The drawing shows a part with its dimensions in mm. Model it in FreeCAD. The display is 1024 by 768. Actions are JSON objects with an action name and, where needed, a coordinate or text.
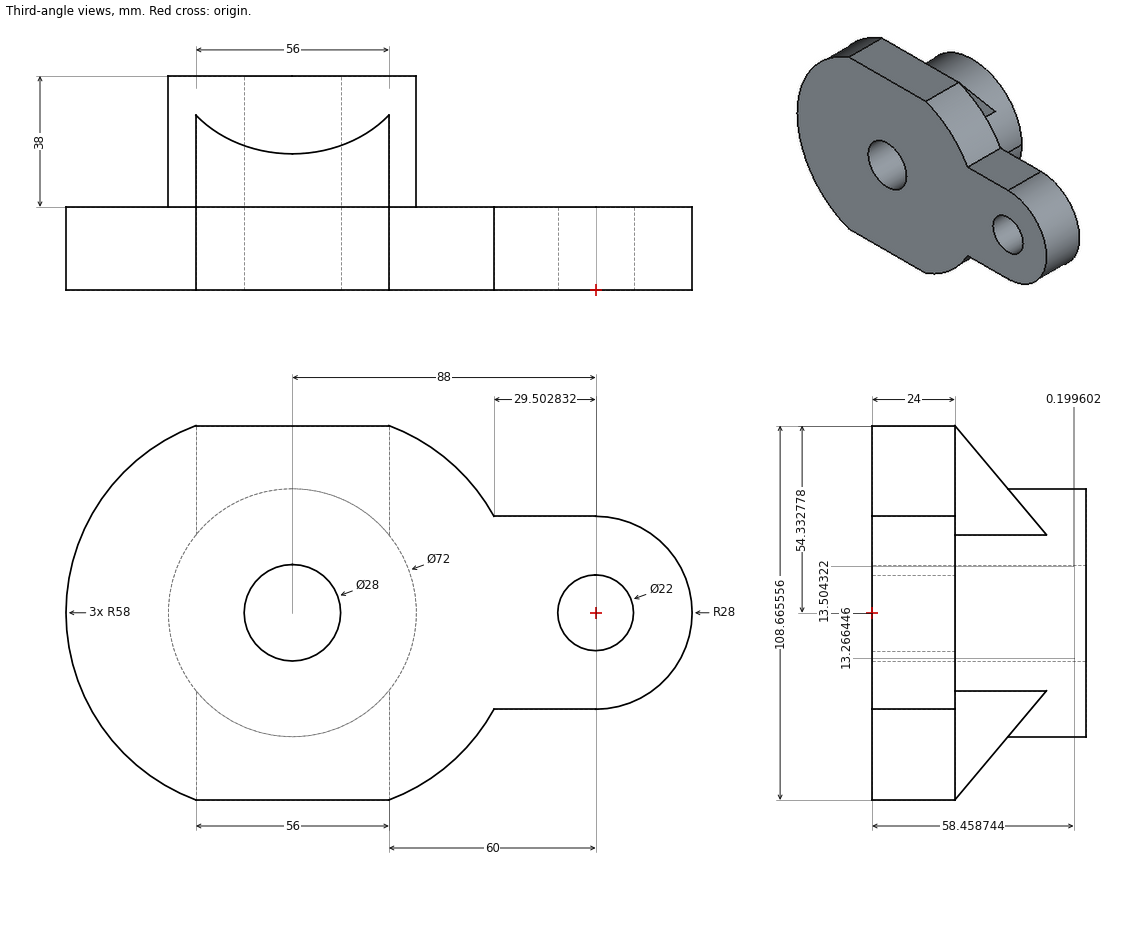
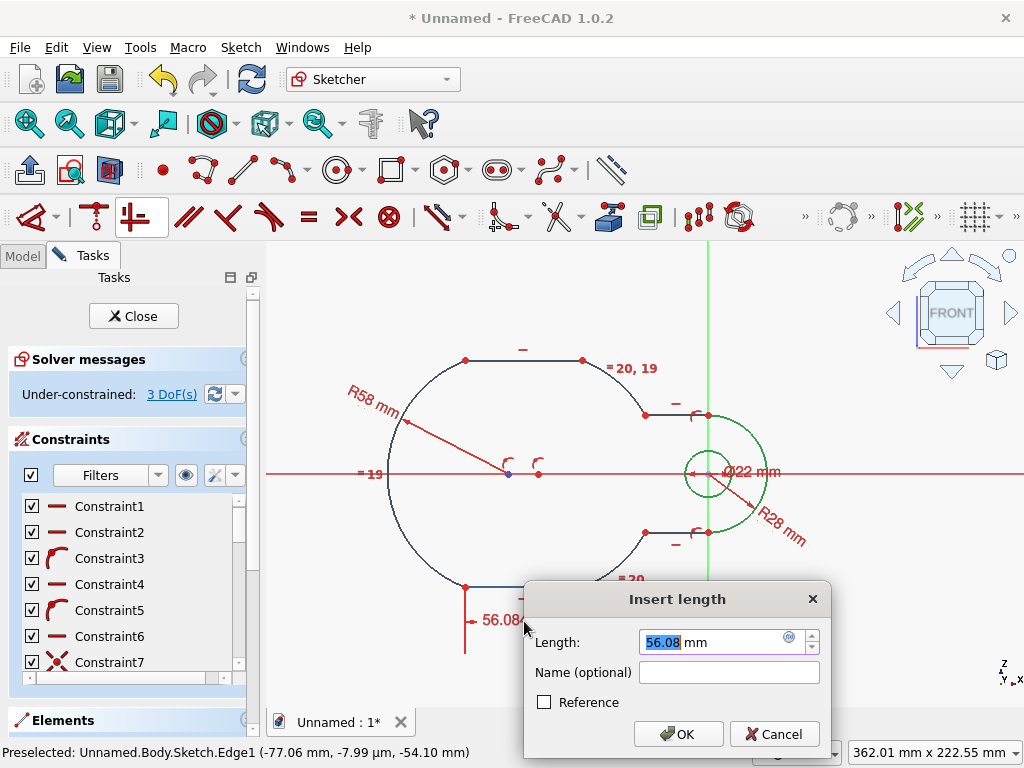
{"action": "type", "text": "56"}
{"action": "key", "text": "Return"}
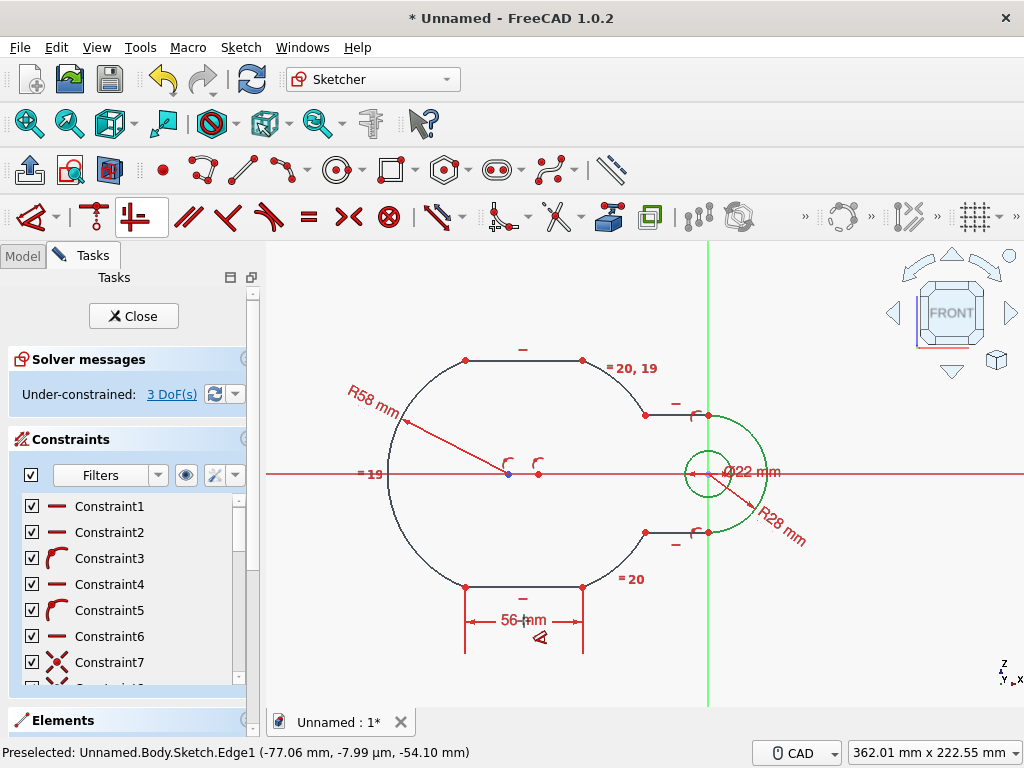
{"action": "left_click", "coordinate": [500, 361]}
{"action": "left_click", "coordinate": [524, 327]}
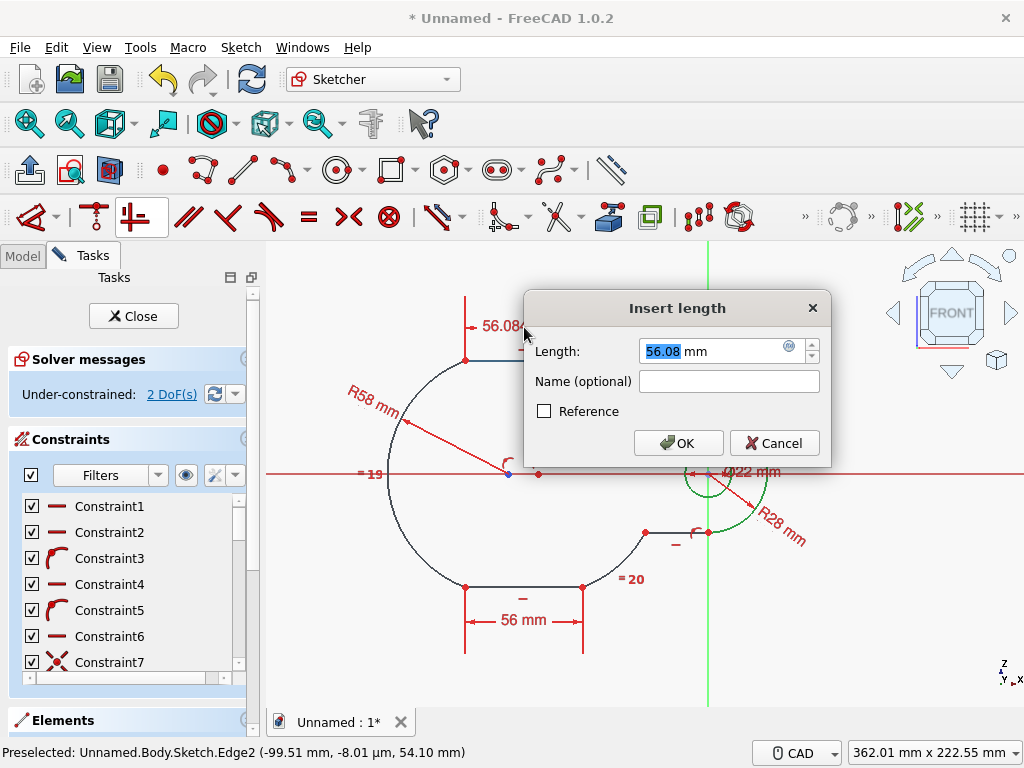
{"action": "type", "text": "56"}
{"action": "key", "text": "Return"}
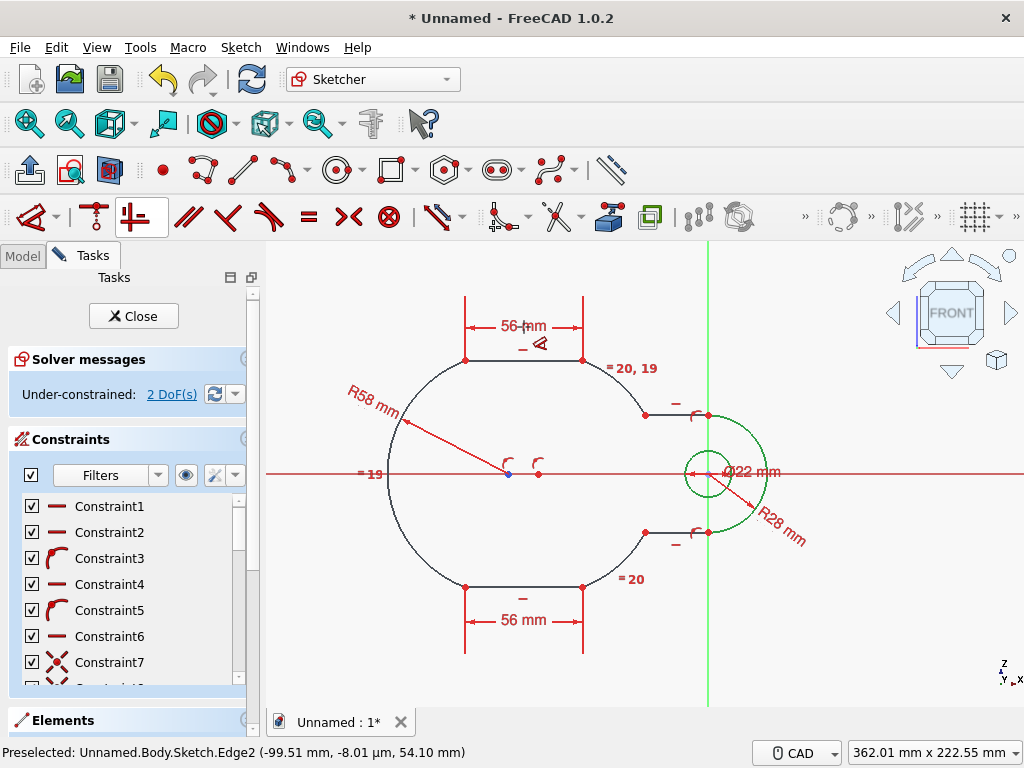
{"action": "left_click", "coordinate": [583, 587]}
{"action": "left_click", "coordinate": [645, 621]}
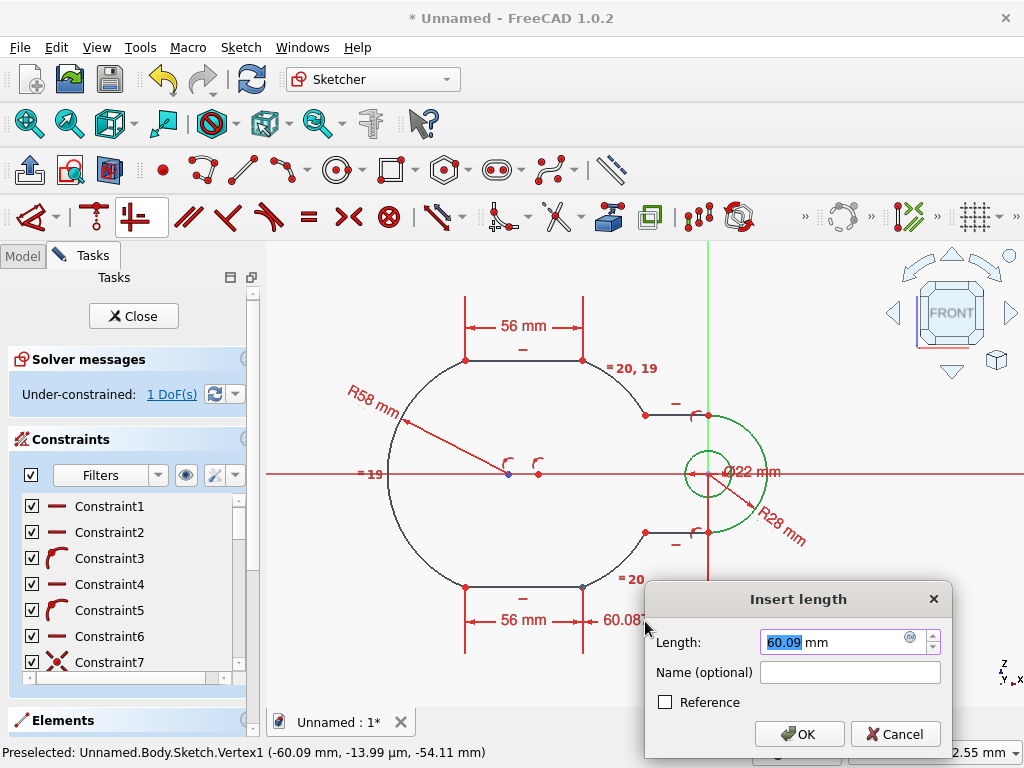
{"action": "type", "text": "60"}
{"action": "key", "text": "Return"}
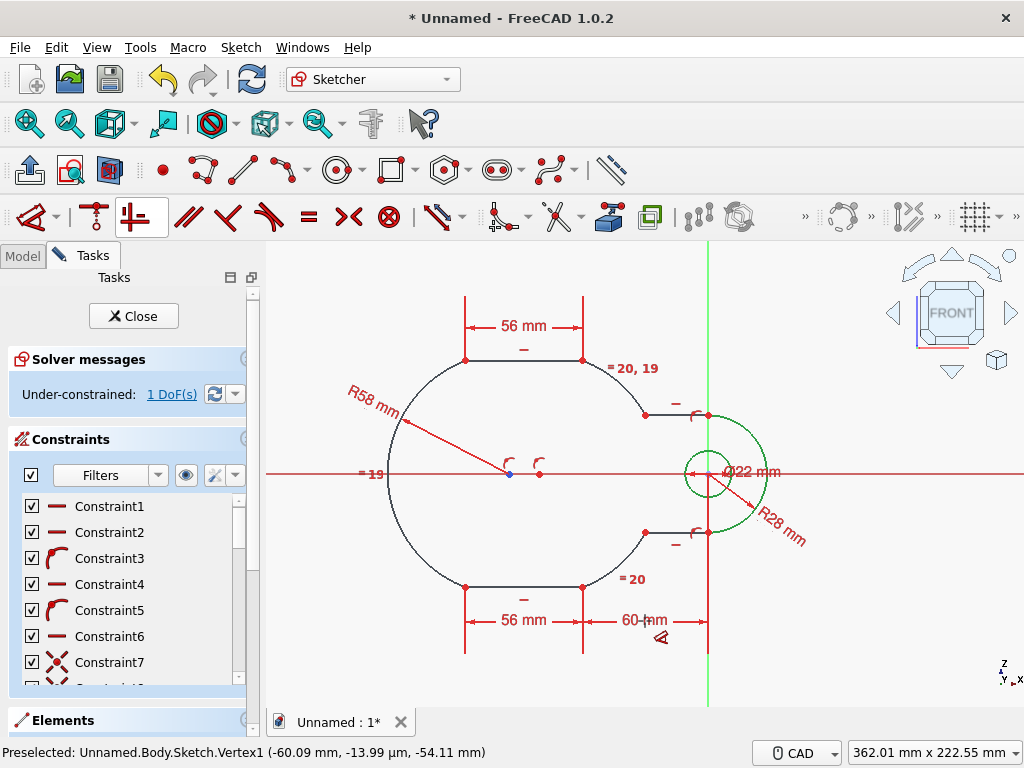
{"action": "left_click", "coordinate": [664, 415]}
{"action": "left_click", "coordinate": [677, 381]}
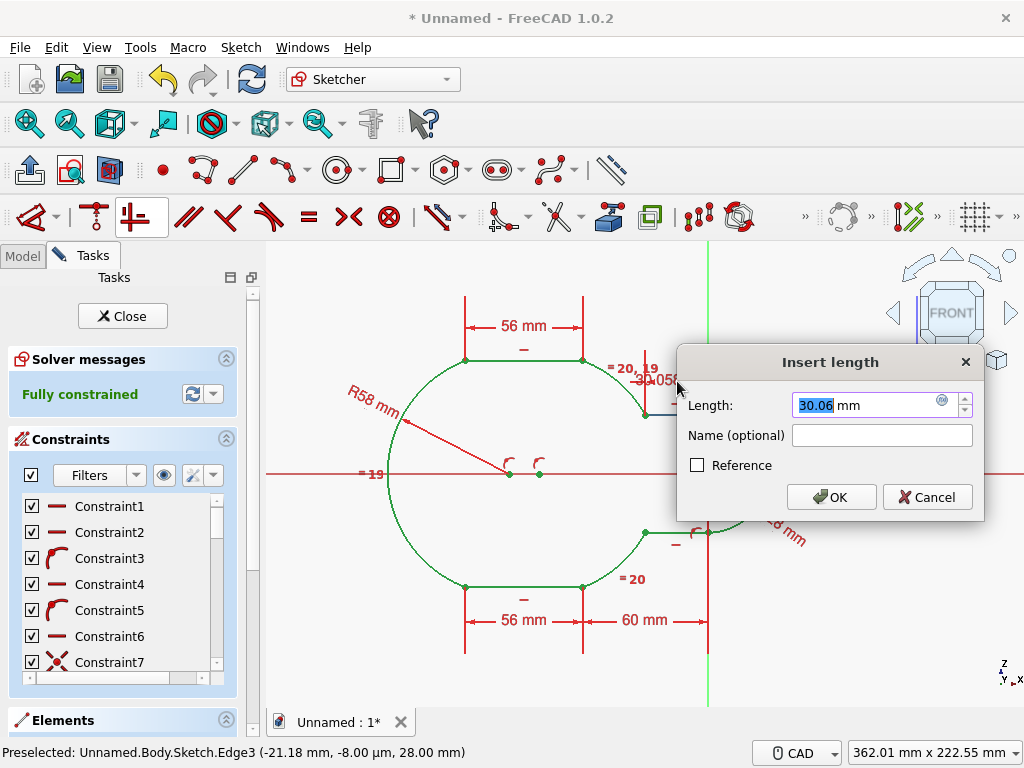
{"action": "type", "text": "29.502832"}
{"action": "key", "text": "Return"}
{"action": "key", "text": "Escape"}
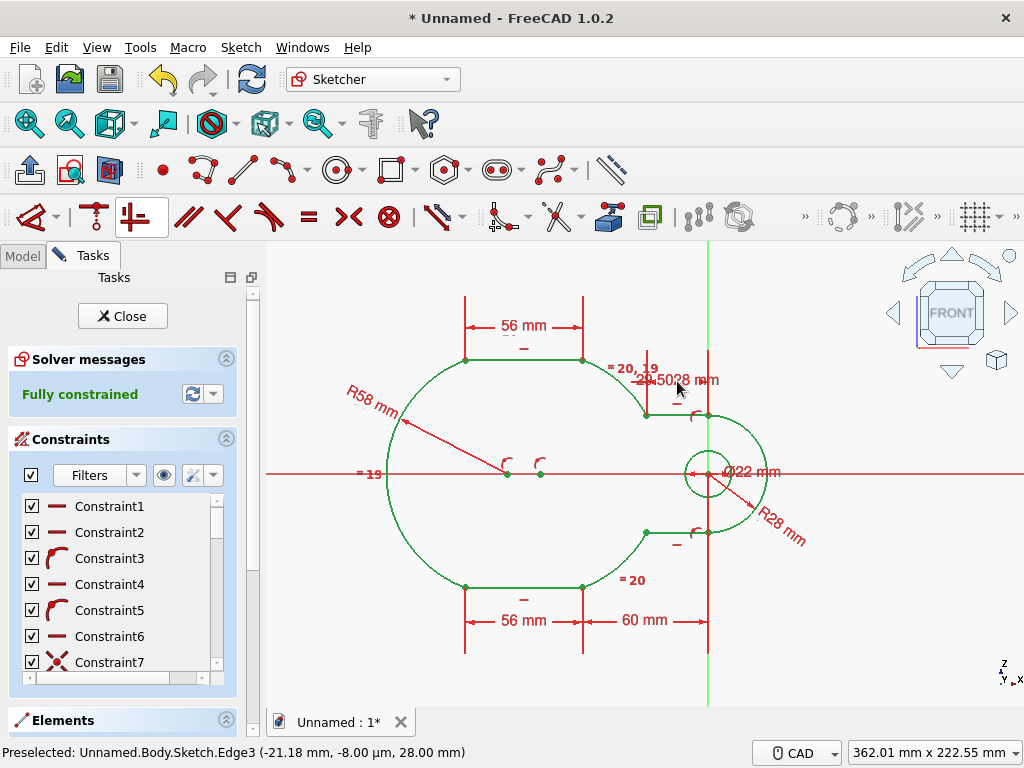
{"action": "left_click", "coordinate": [123, 316]}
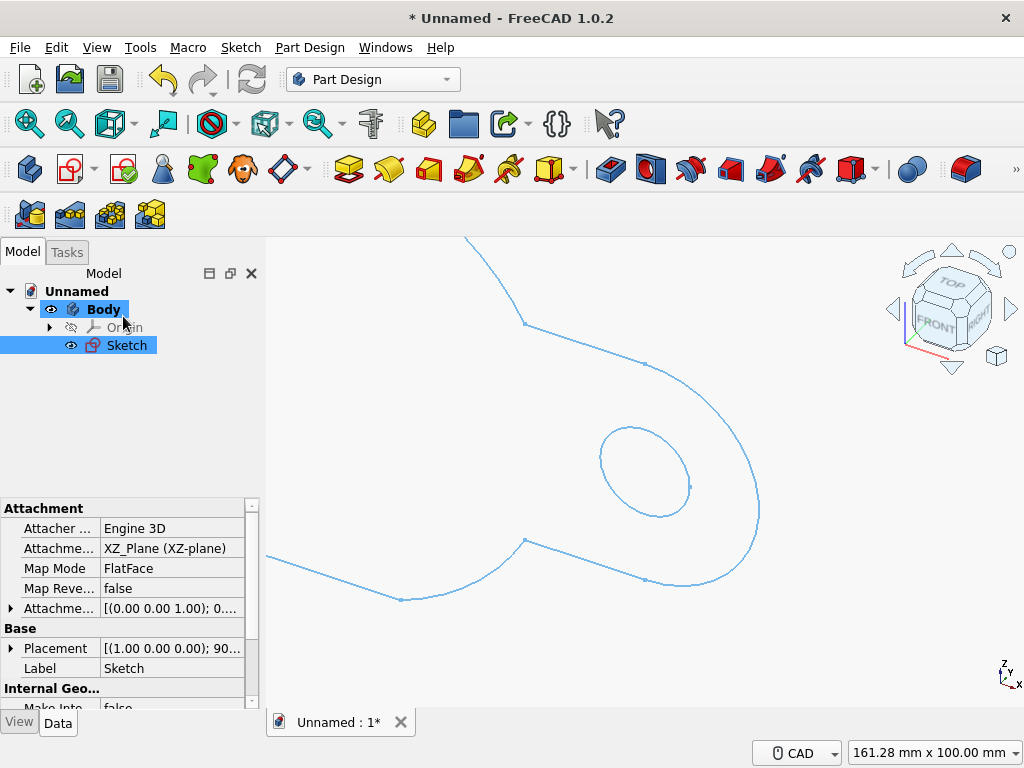
{"action": "left_click", "coordinate": [350, 170]}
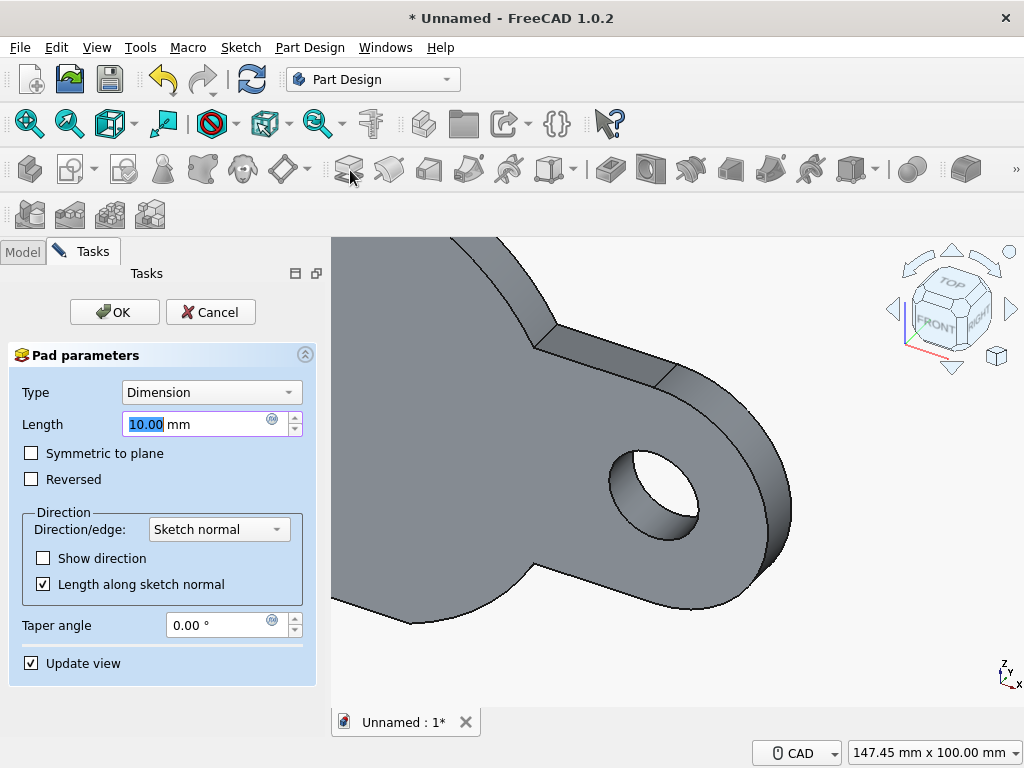
{"action": "type", "text": "24"}
{"action": "key", "text": "Tab"}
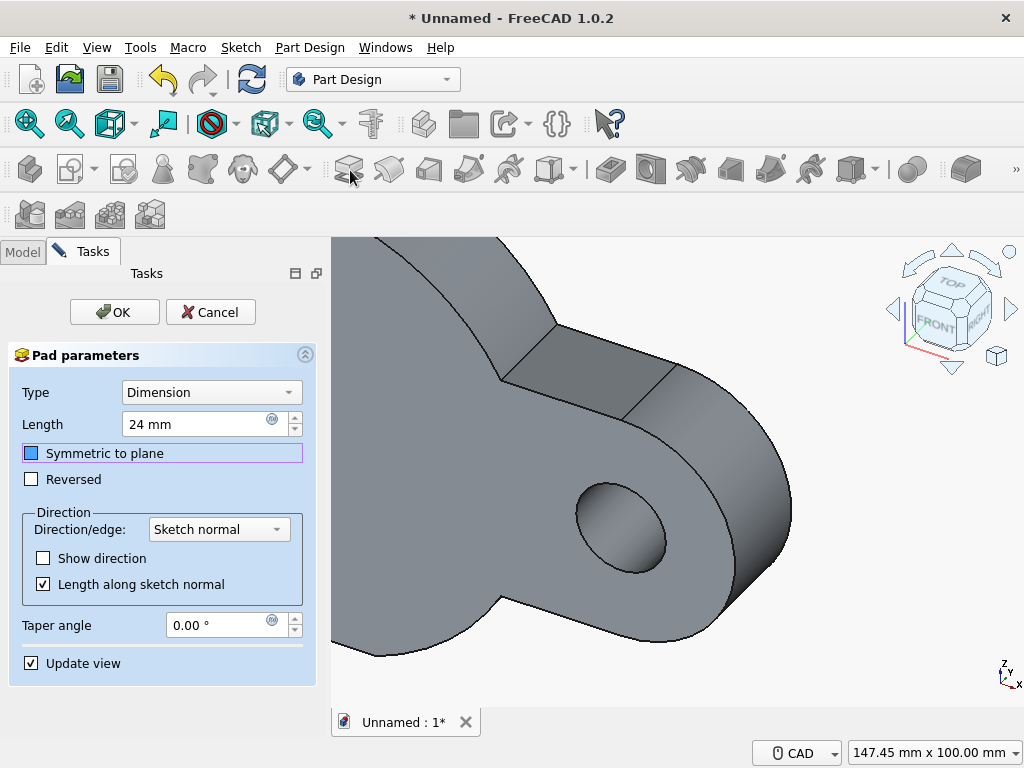
{"action": "left_click", "coordinate": [30, 479]}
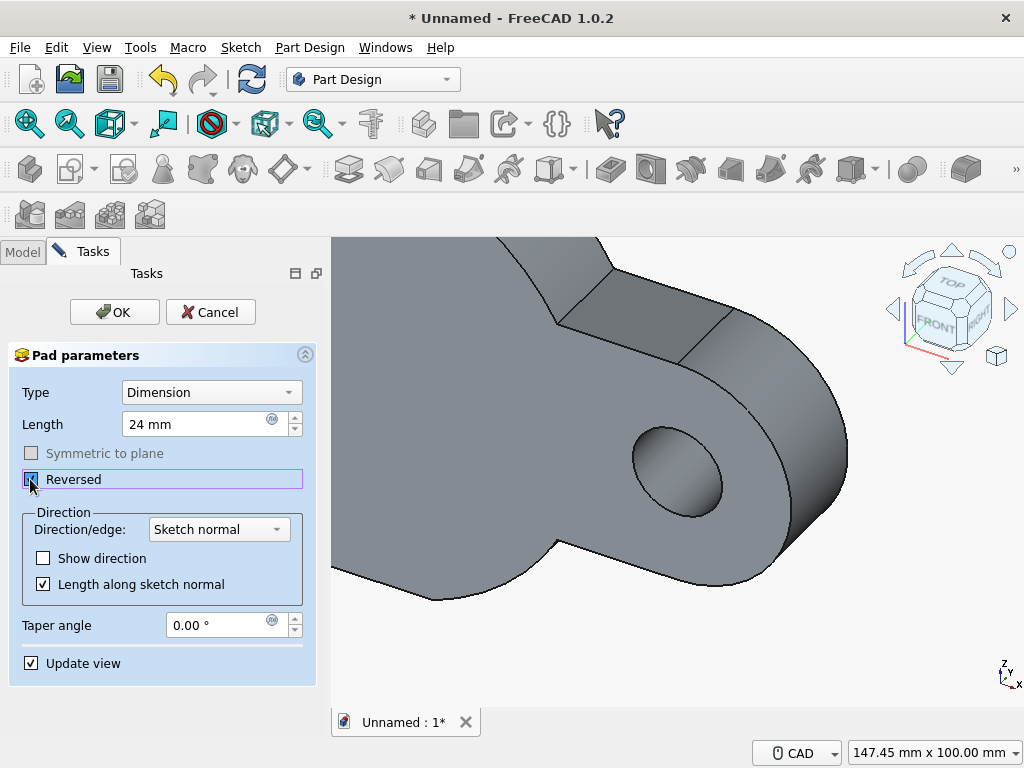
{"action": "left_click", "coordinate": [115, 312]}